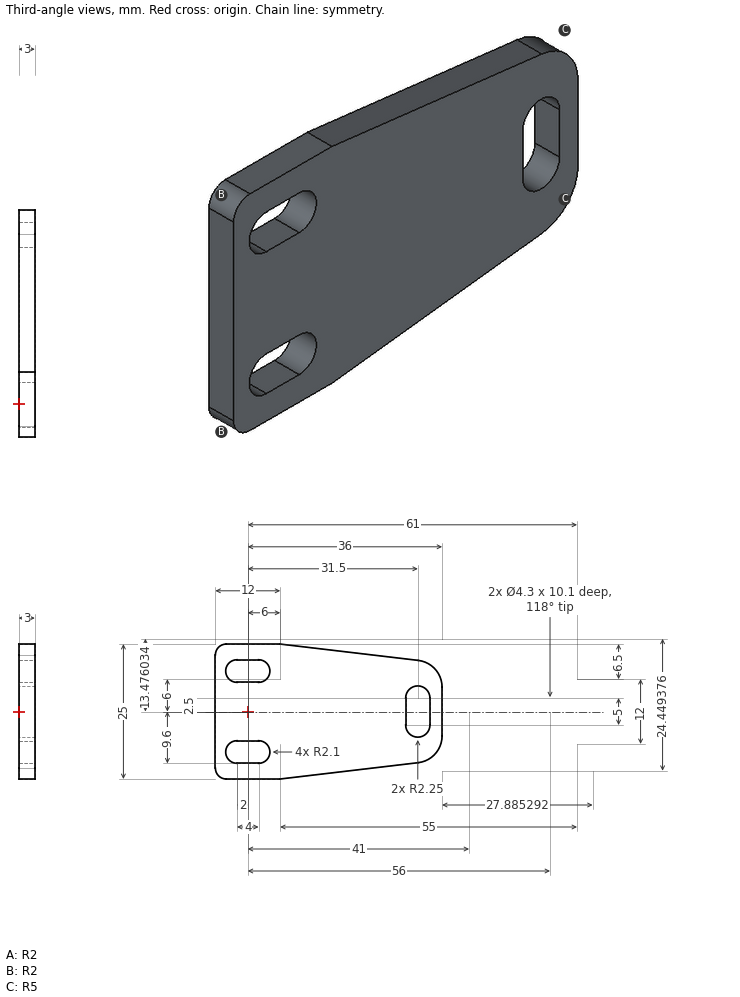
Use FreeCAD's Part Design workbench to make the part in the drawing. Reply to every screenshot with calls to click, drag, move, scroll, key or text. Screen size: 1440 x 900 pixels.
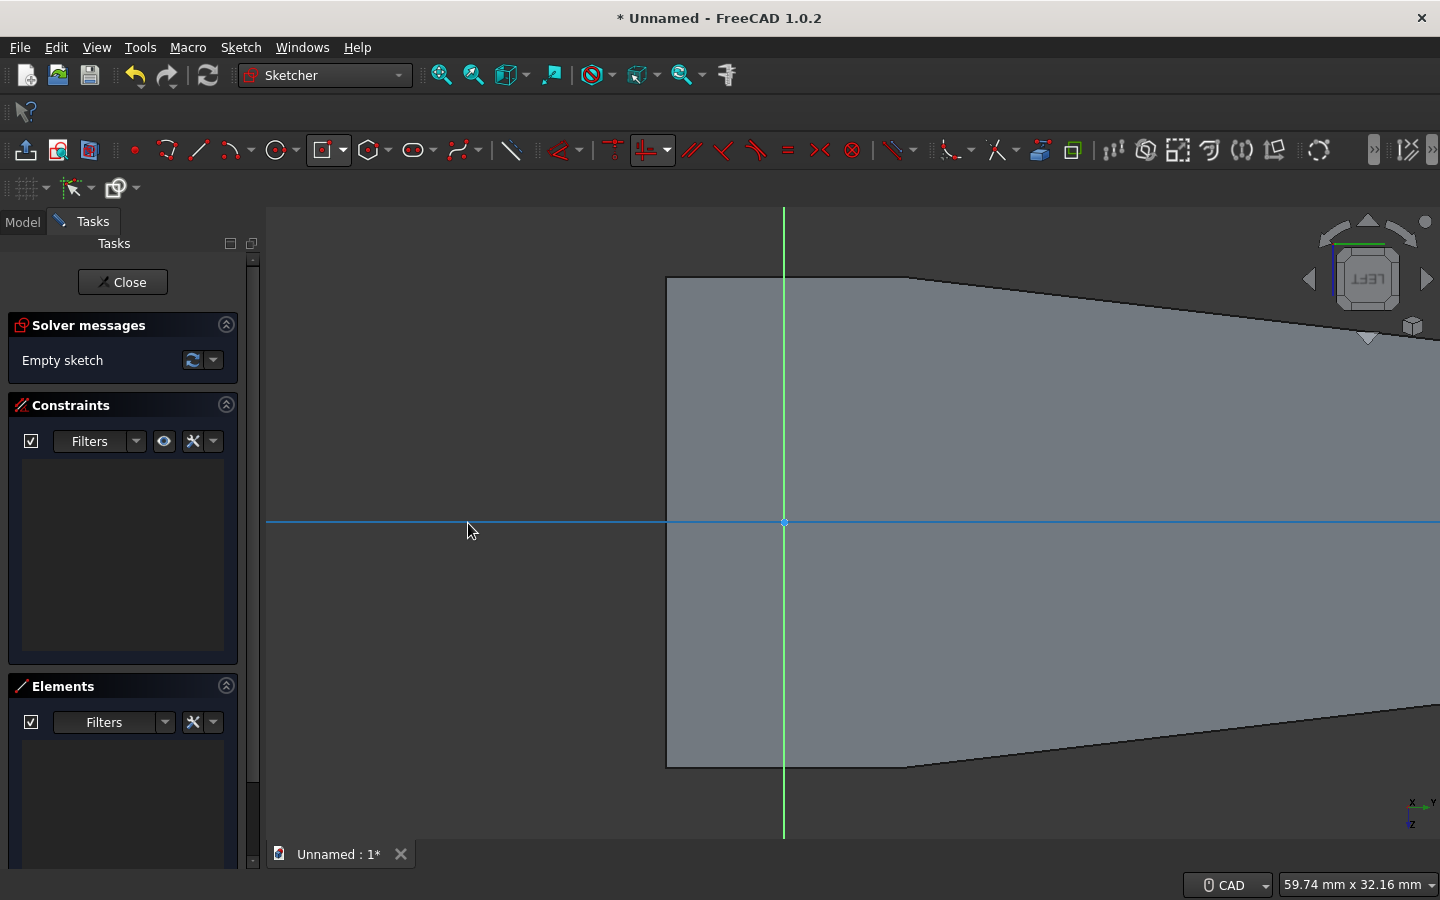
click(414, 150)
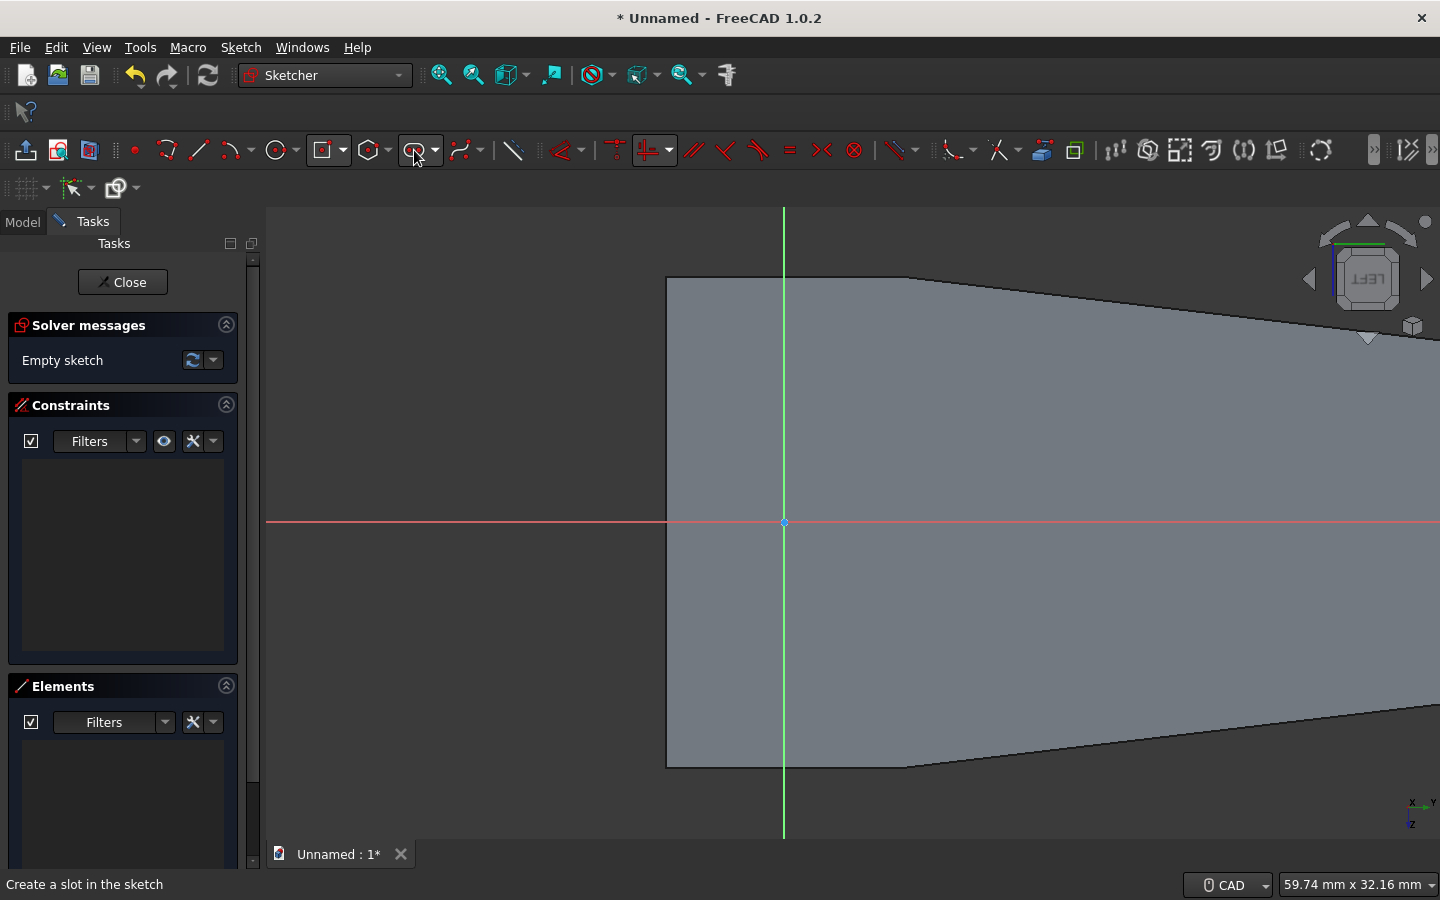
click(745, 375)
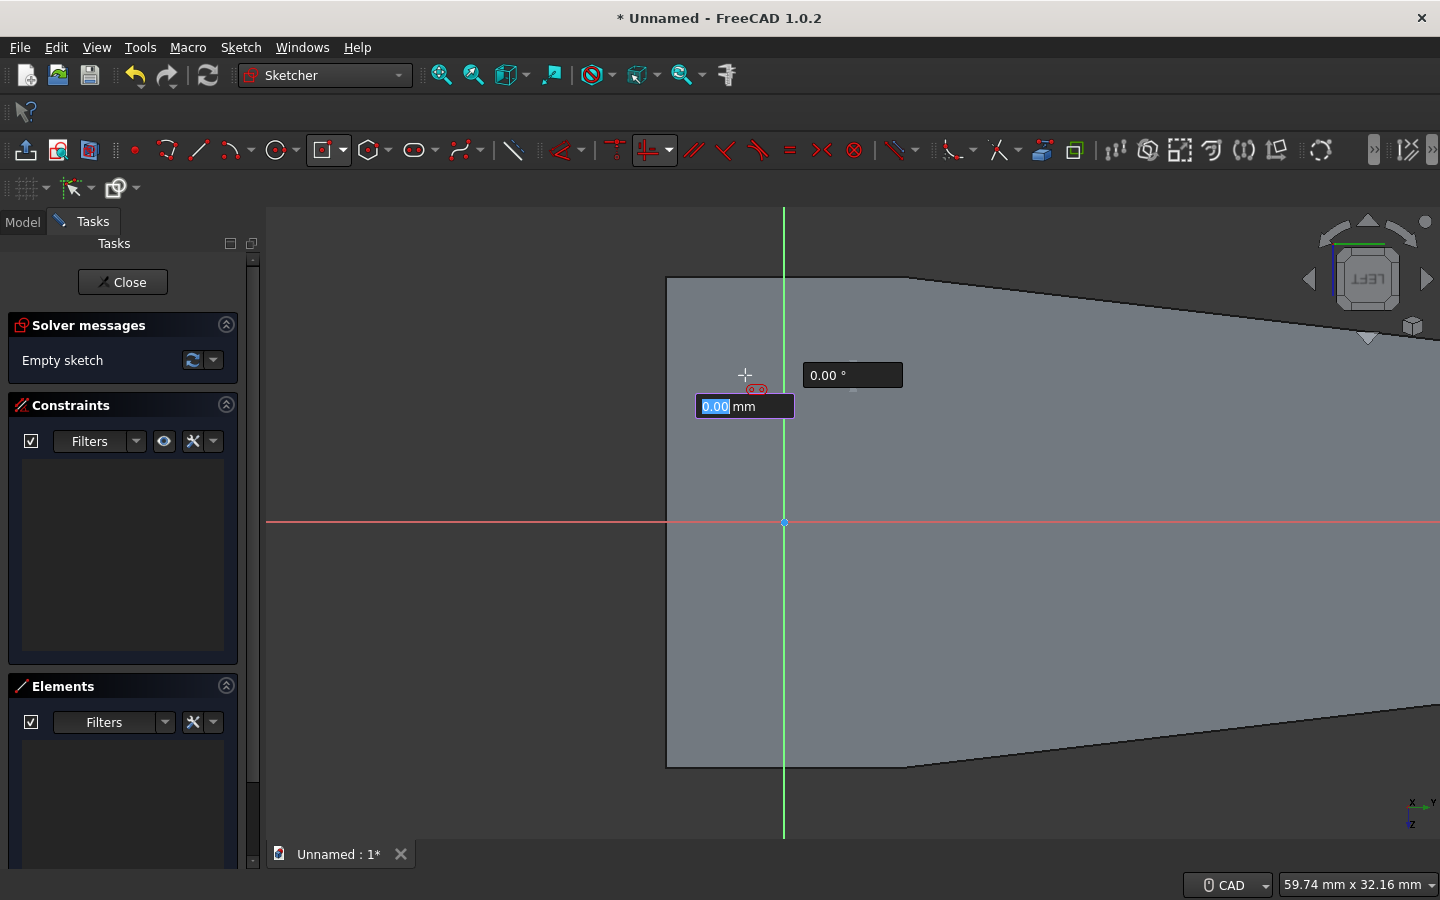
click(824, 375)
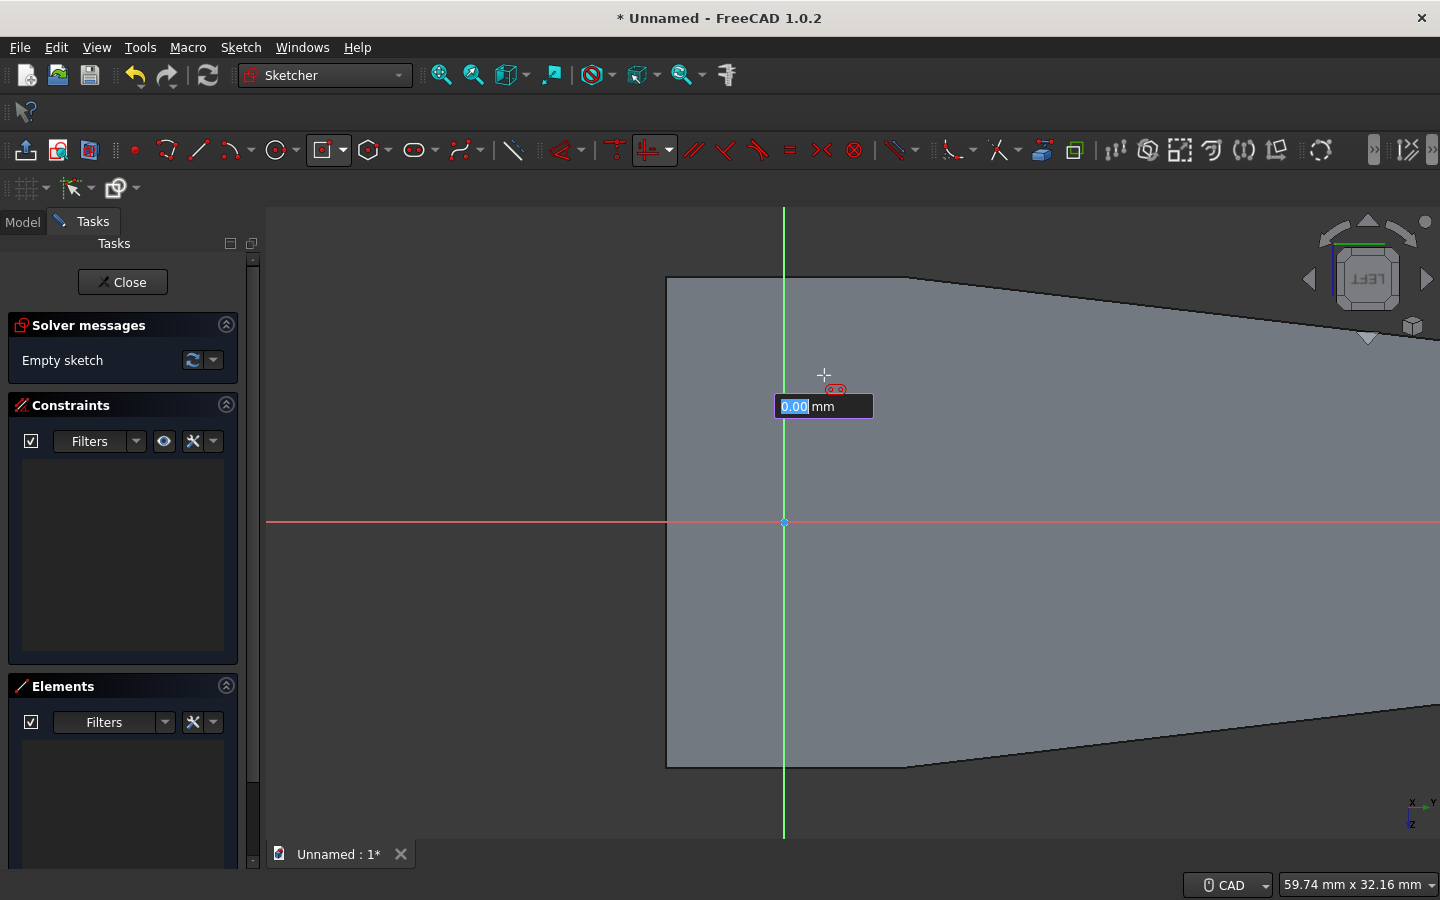
scroll(772, 416, up, 2)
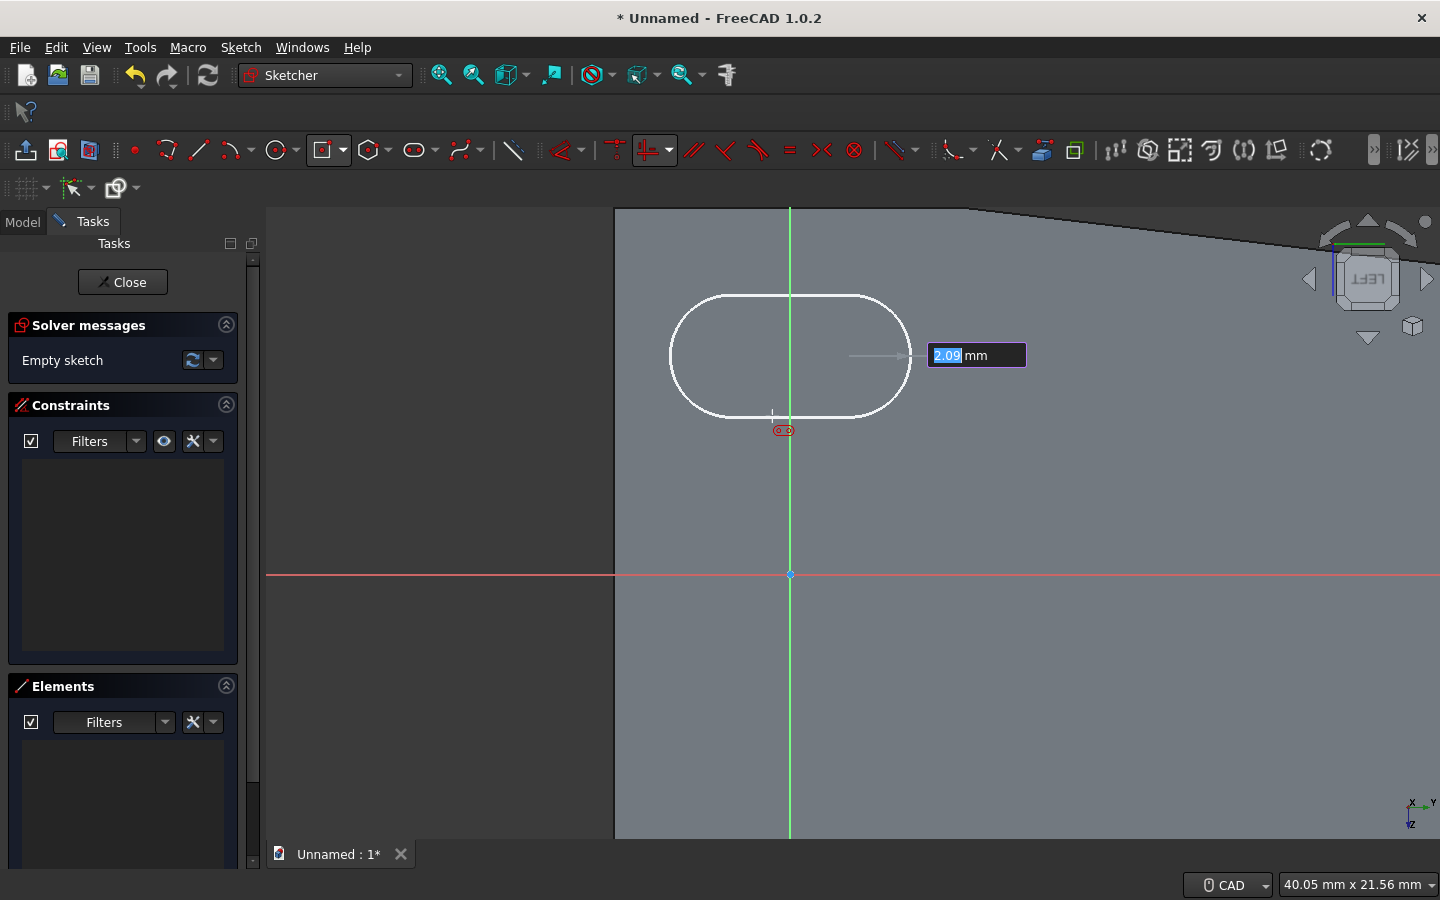
click(772, 416)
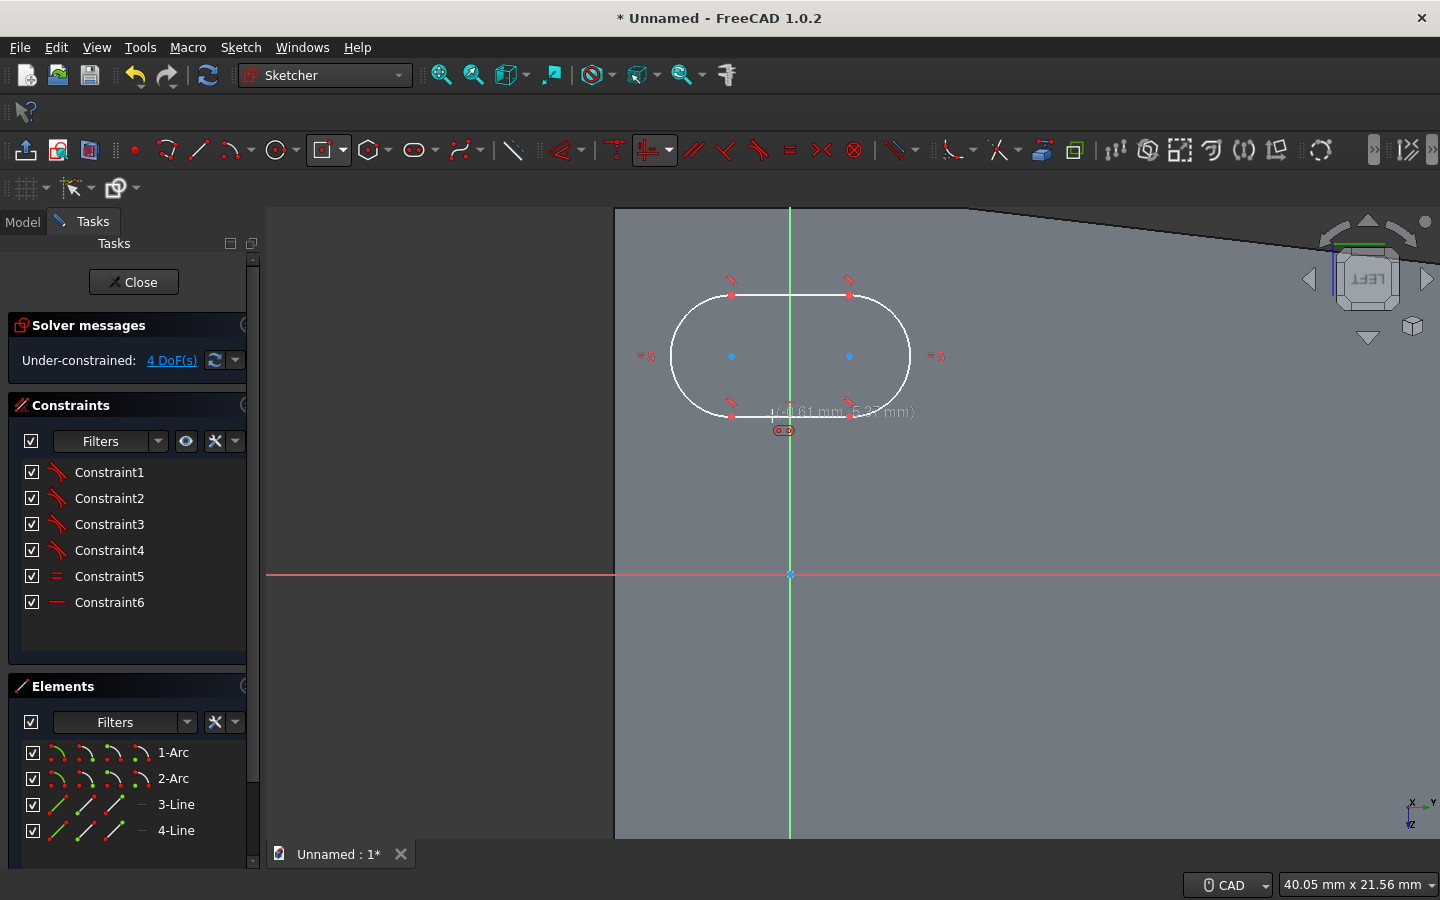
click(731, 794)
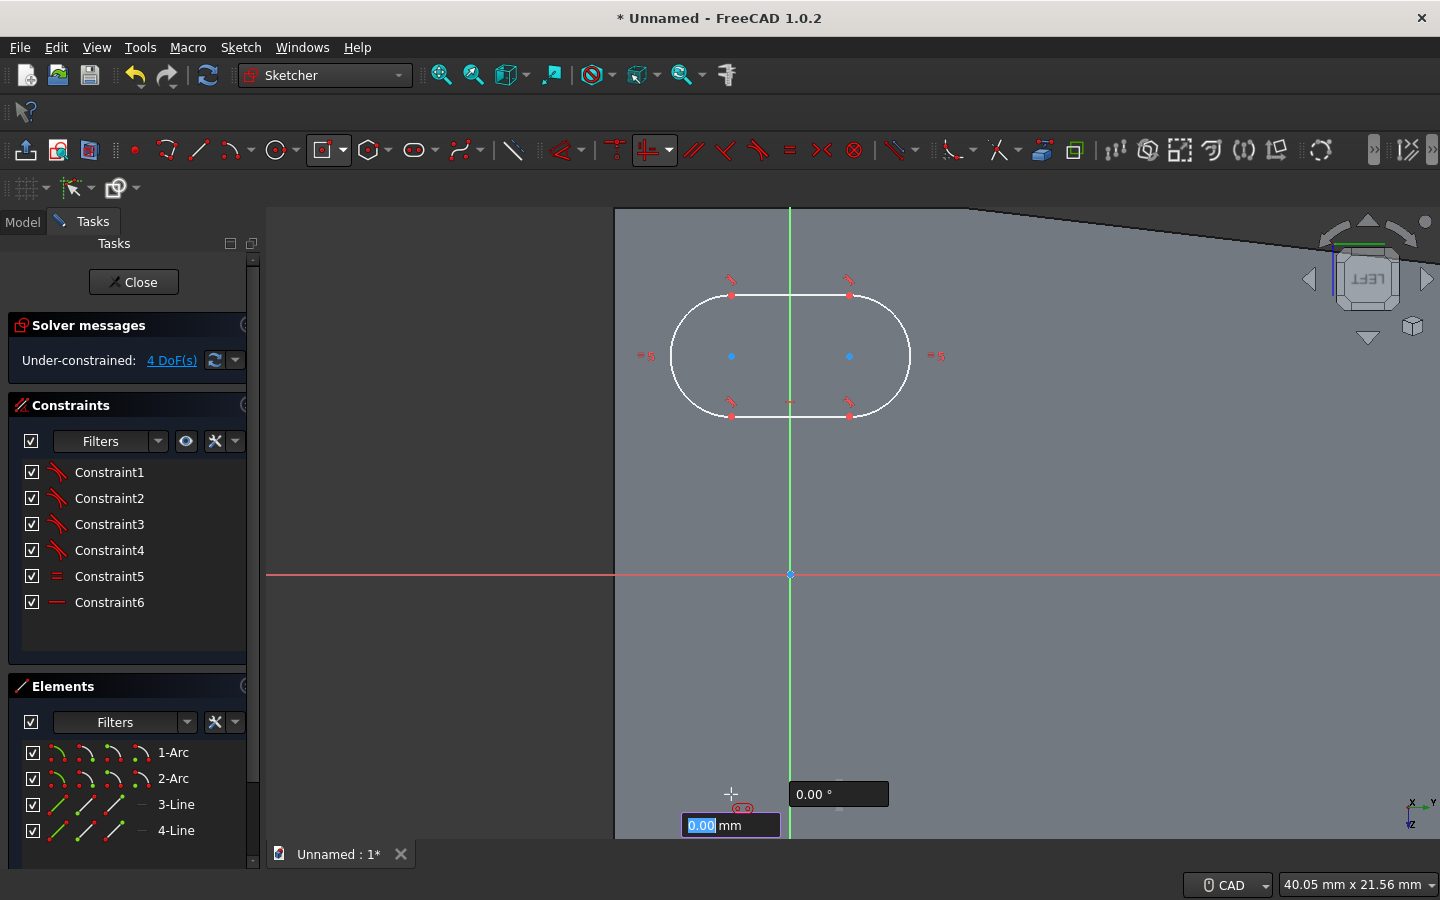
click(849, 794)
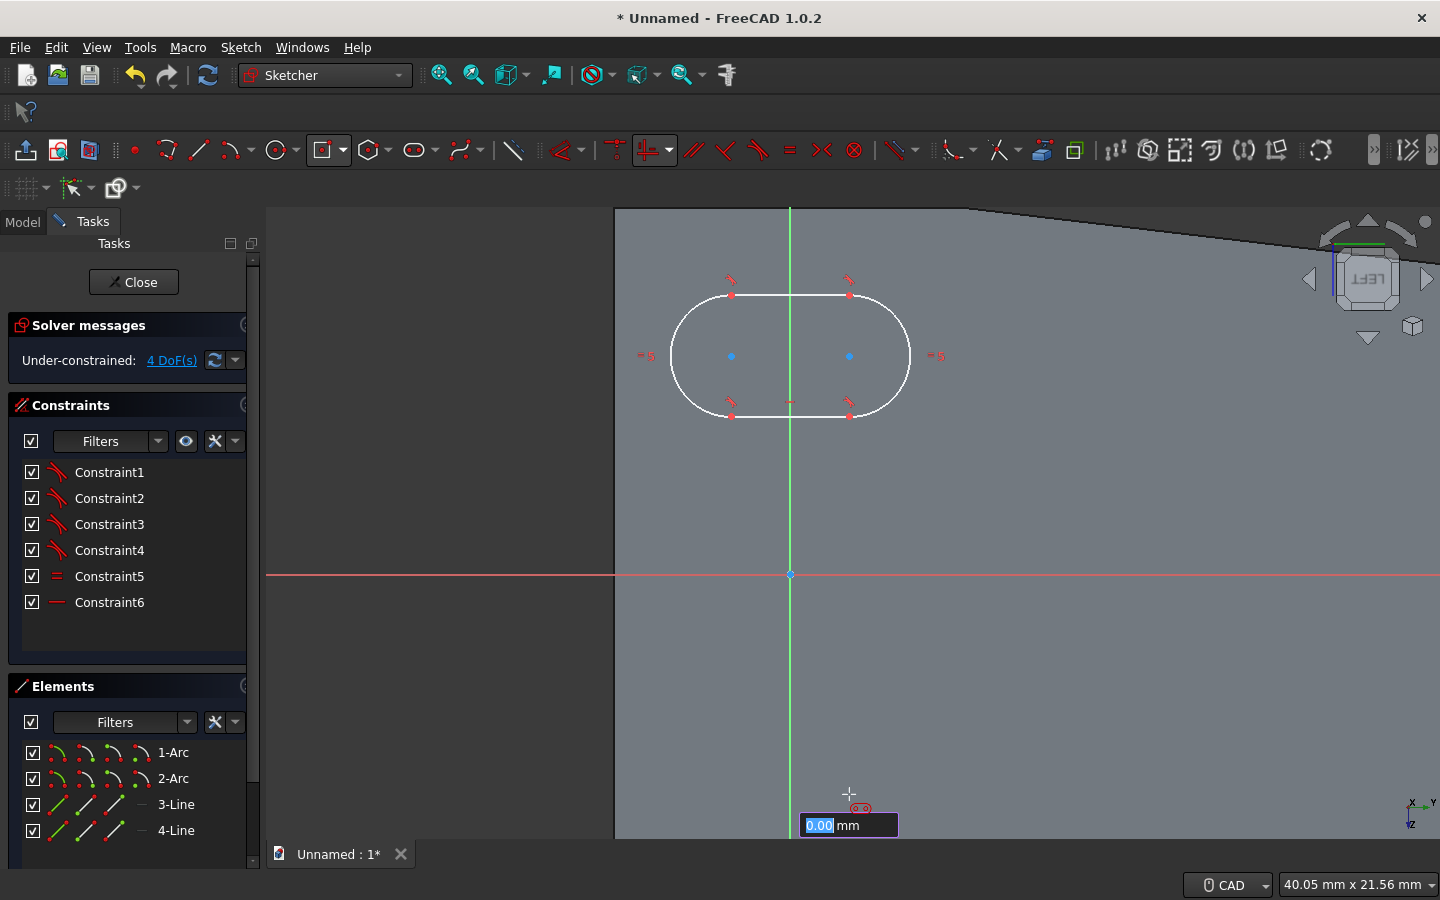
click(808, 733)
key(Escape)